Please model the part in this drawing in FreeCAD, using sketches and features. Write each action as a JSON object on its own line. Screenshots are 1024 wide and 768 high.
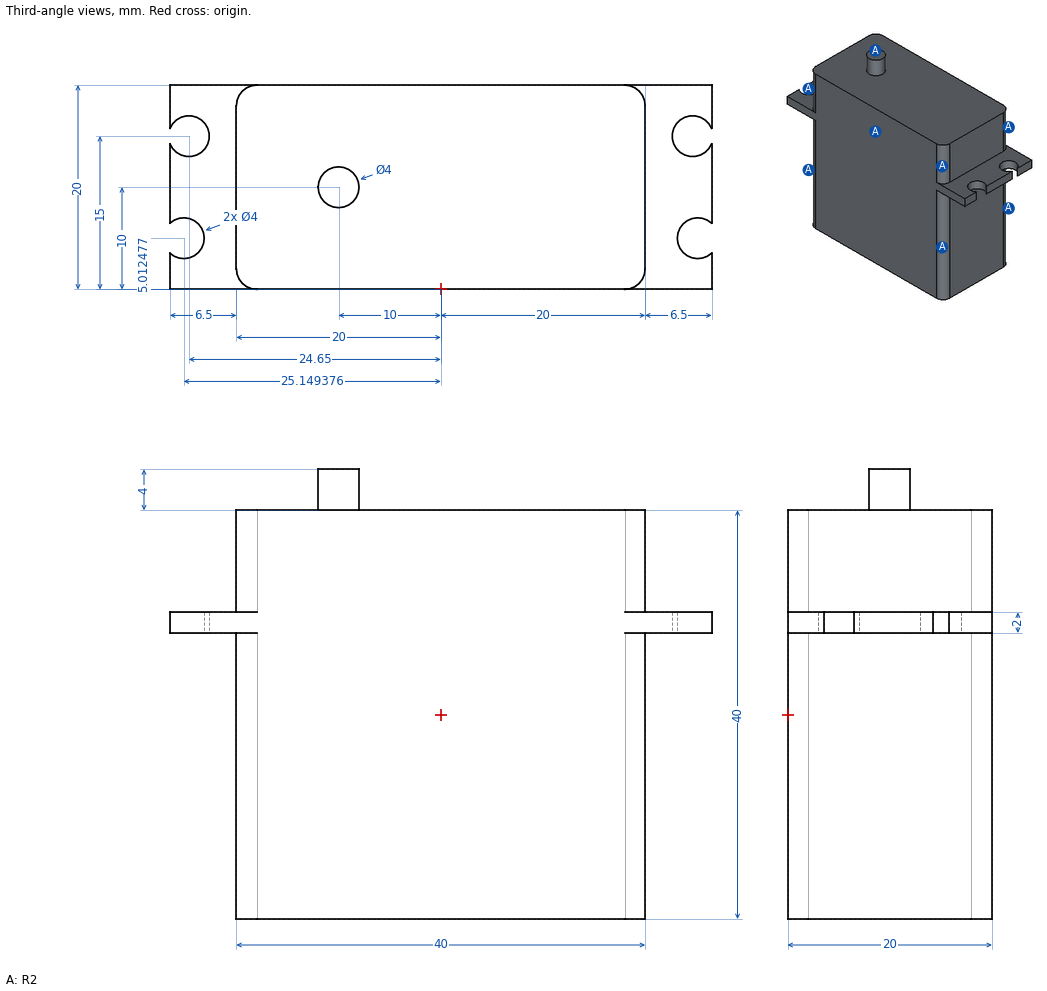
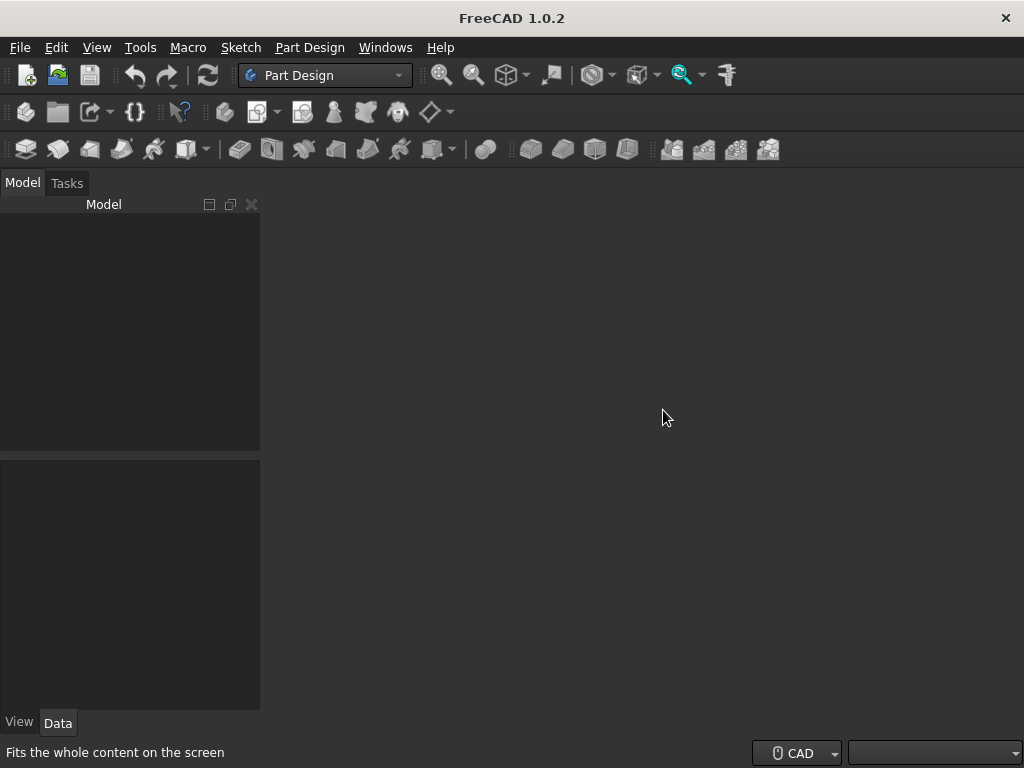
{"action": "key", "text": "ctrl+n"}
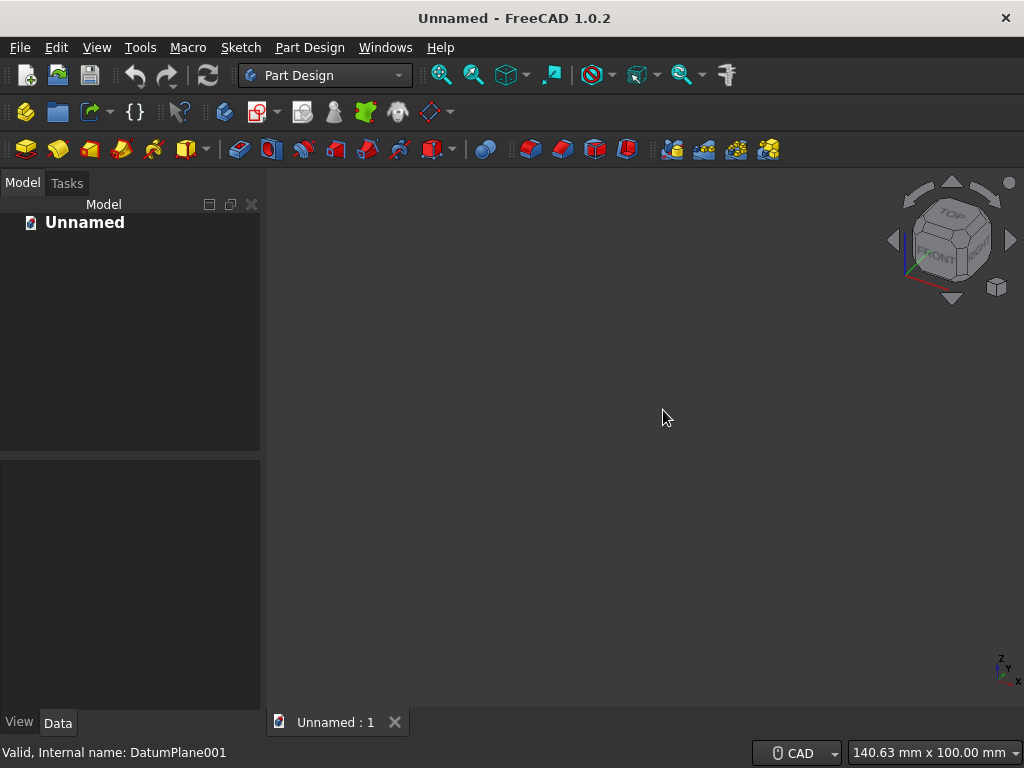
{"action": "left_click", "coordinate": [258, 112]}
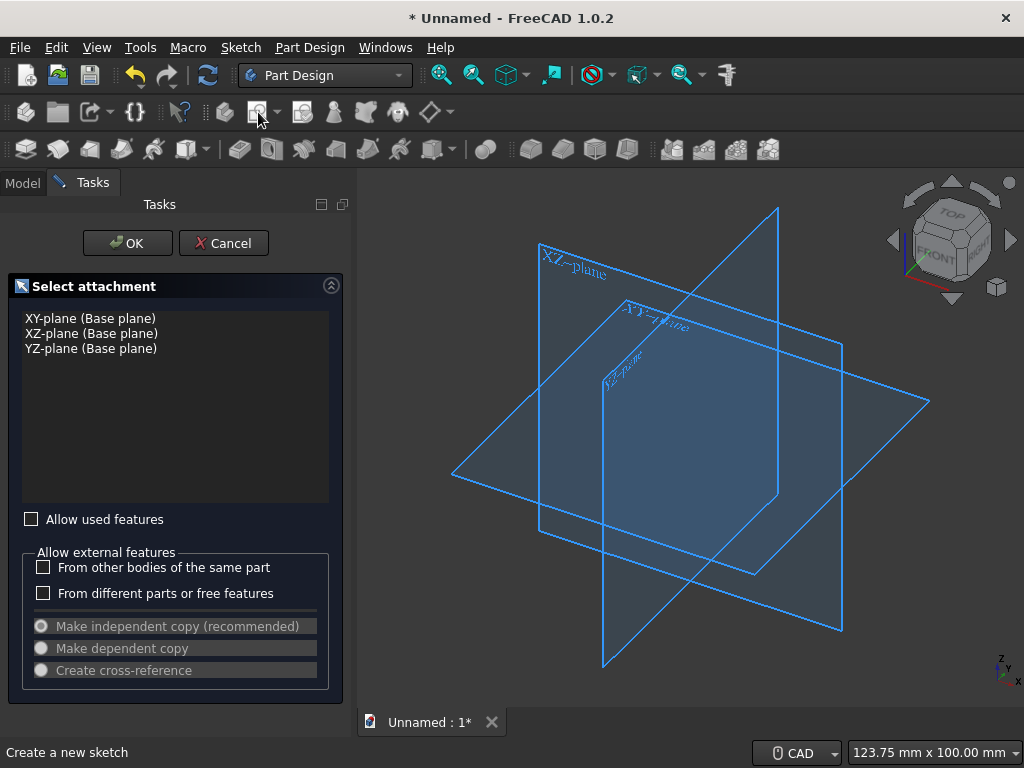
{"action": "left_click", "coordinate": [82, 334]}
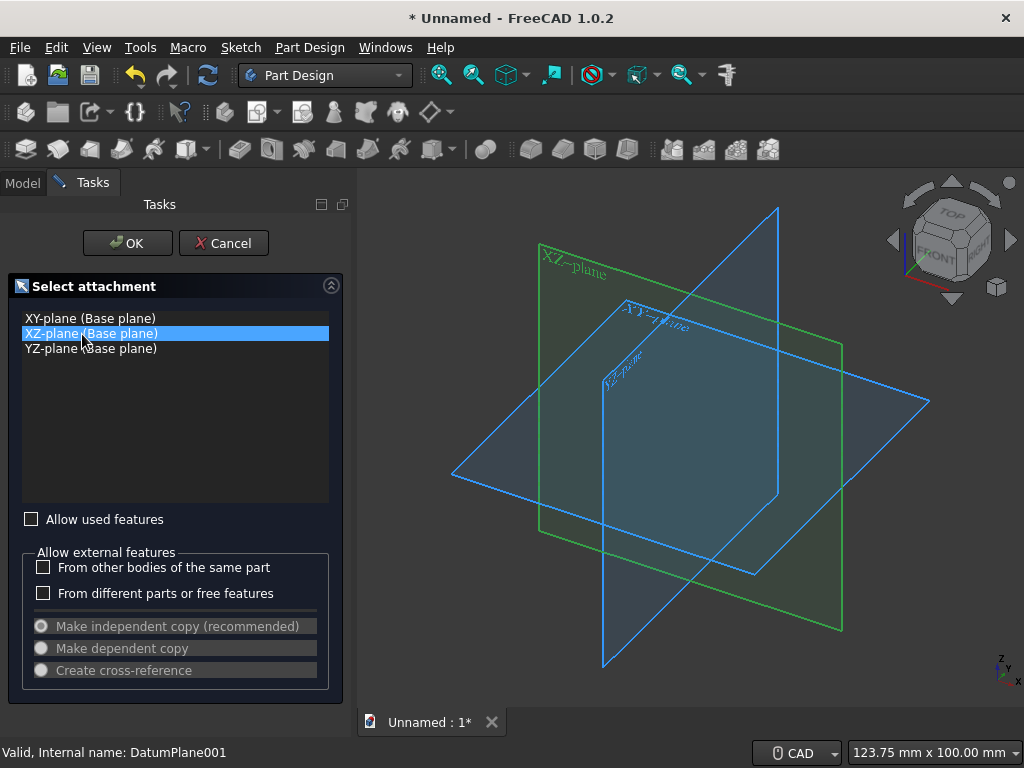
{"action": "left_click", "coordinate": [128, 243]}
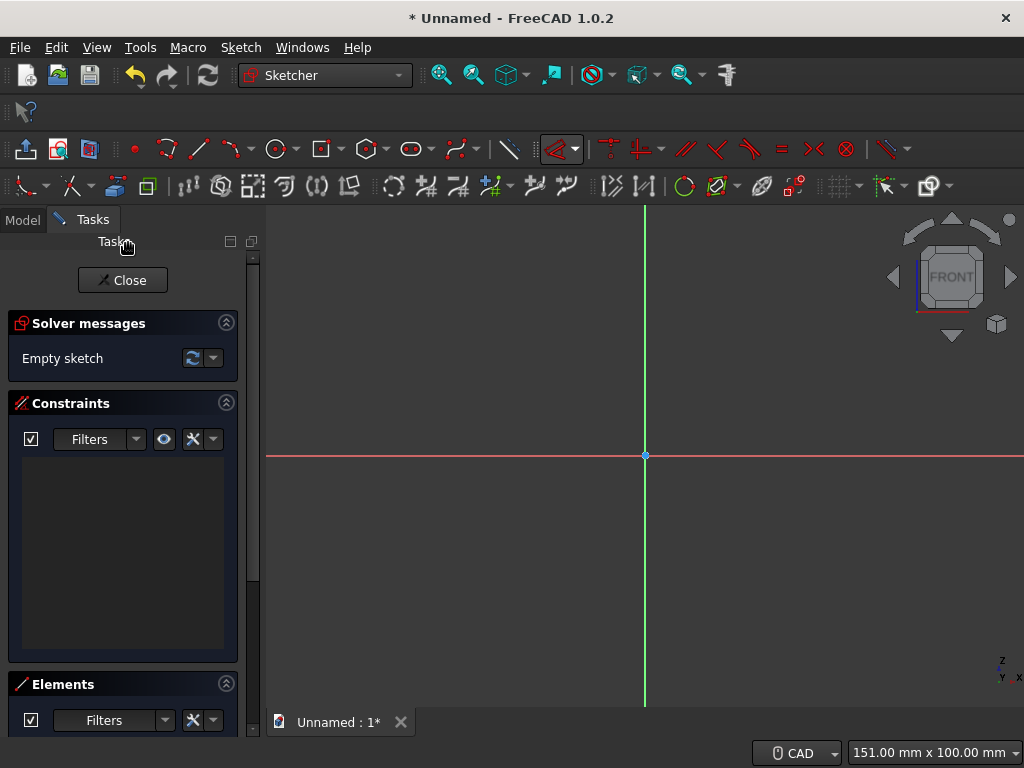
{"action": "scroll", "coordinate": [784, 456], "scroll_direction": "up", "scroll_amount": 2}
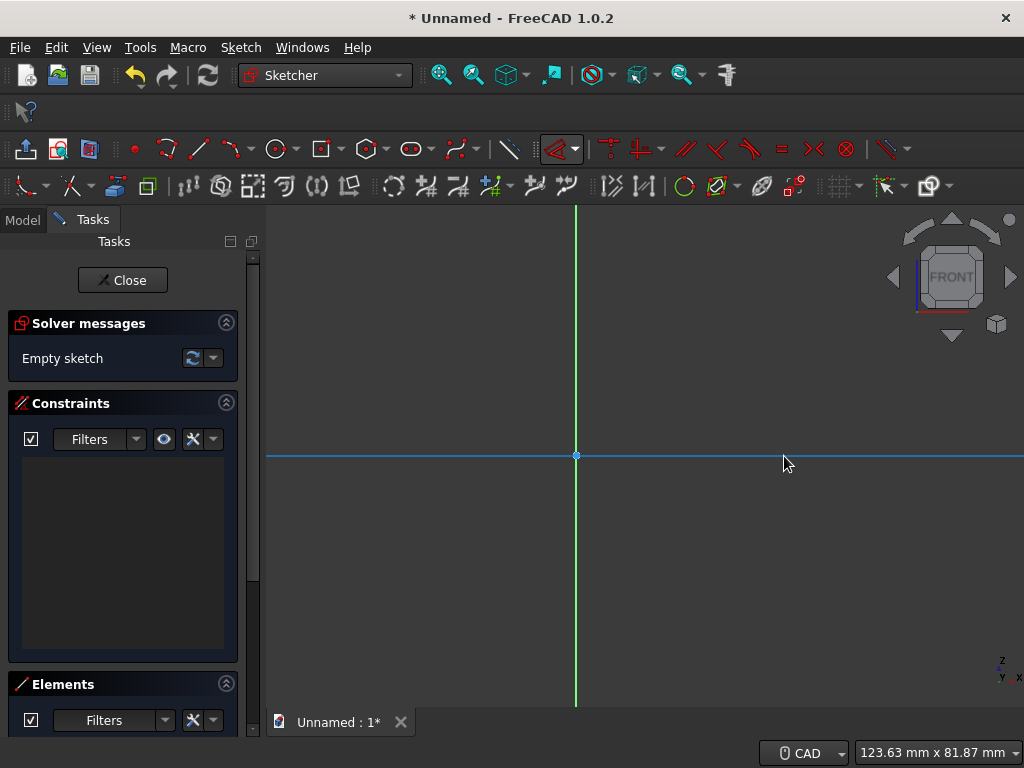
{"action": "left_click", "coordinate": [322, 150]}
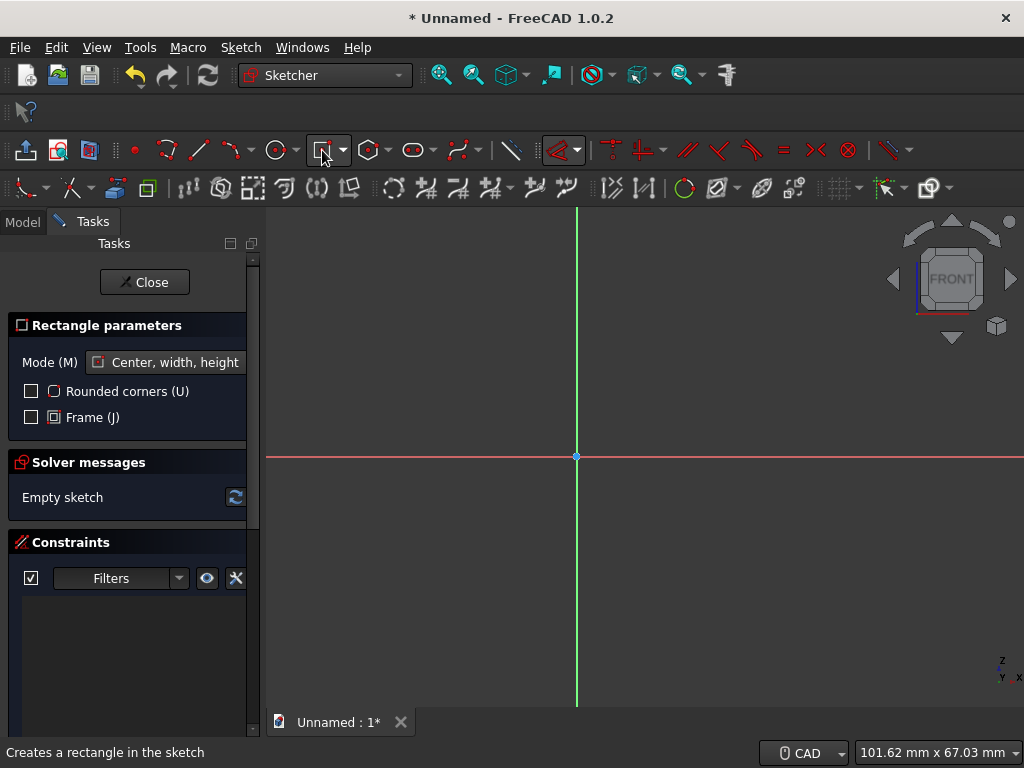
{"action": "left_click", "coordinate": [577, 457]}
{"action": "left_click", "coordinate": [726, 308]}
{"action": "key", "text": "Escape"}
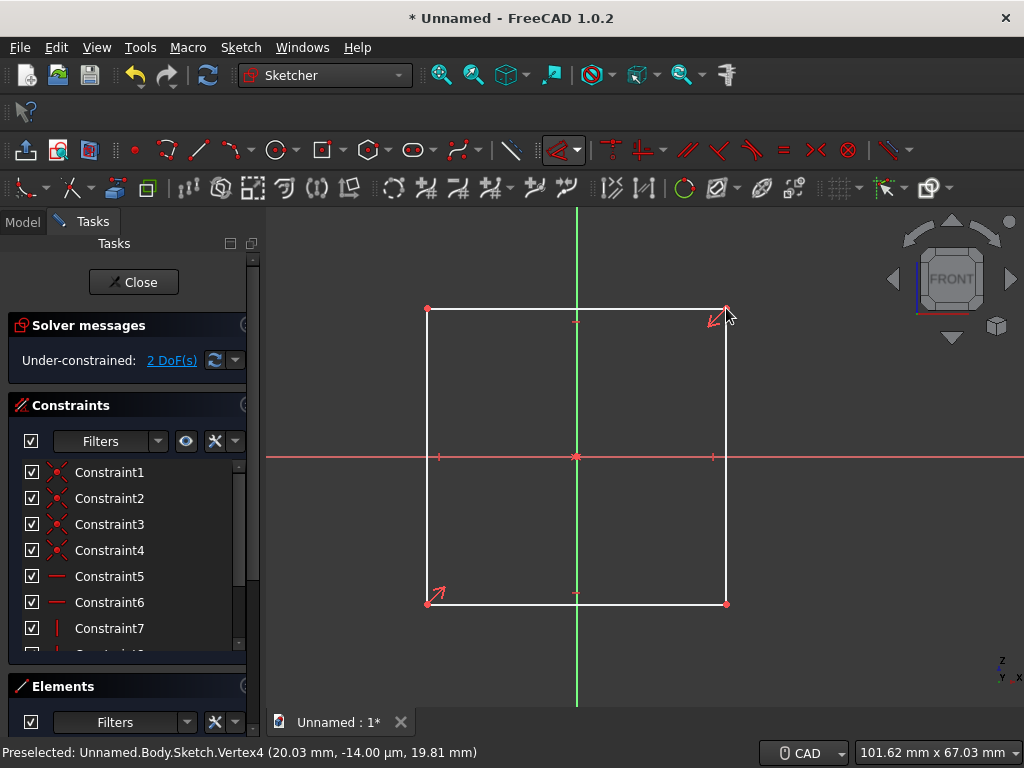
{"action": "left_click", "coordinate": [517, 605]}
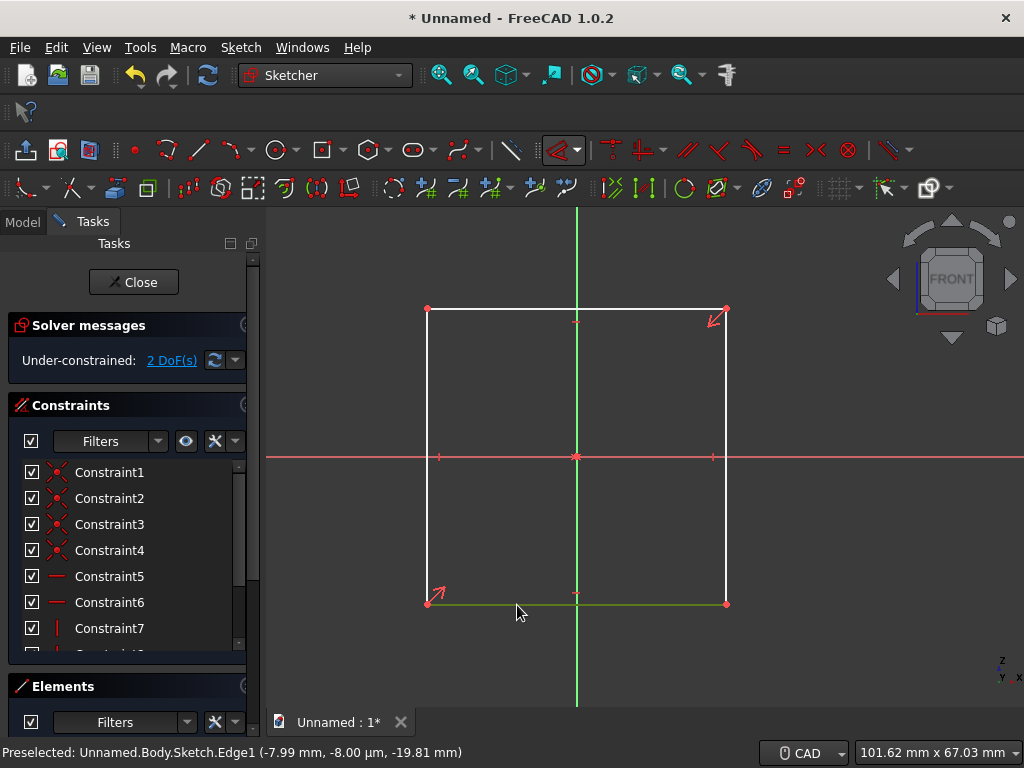
{"action": "key", "text": "l"}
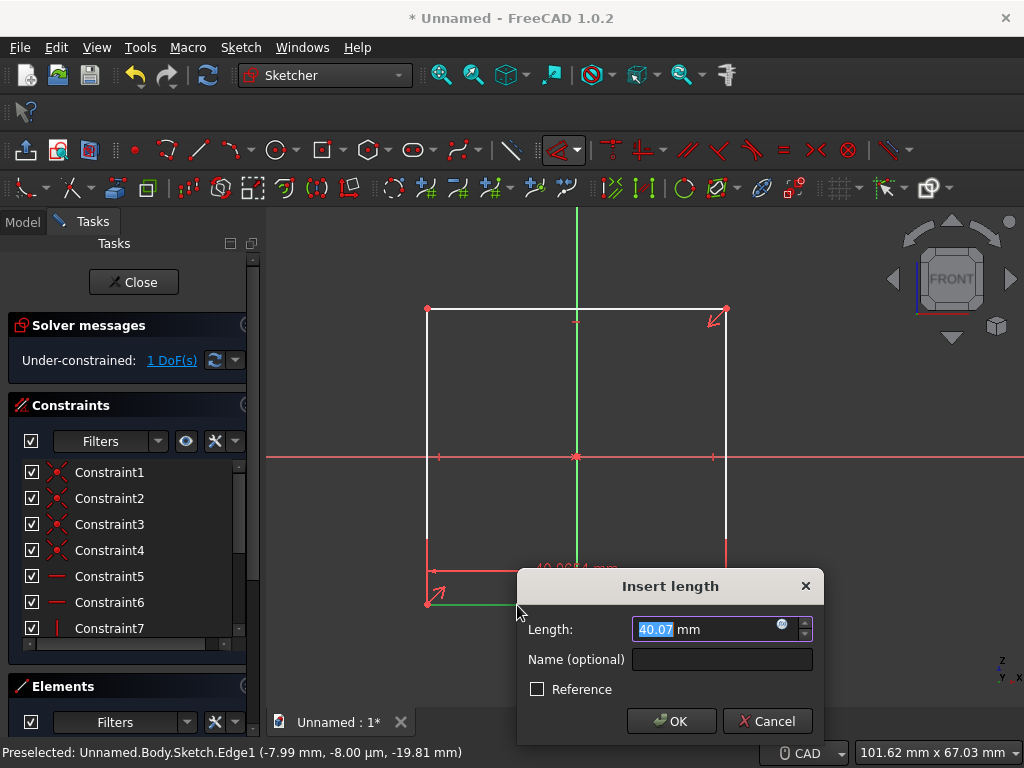
{"action": "type", "text": "40"}
{"action": "key", "text": "Return"}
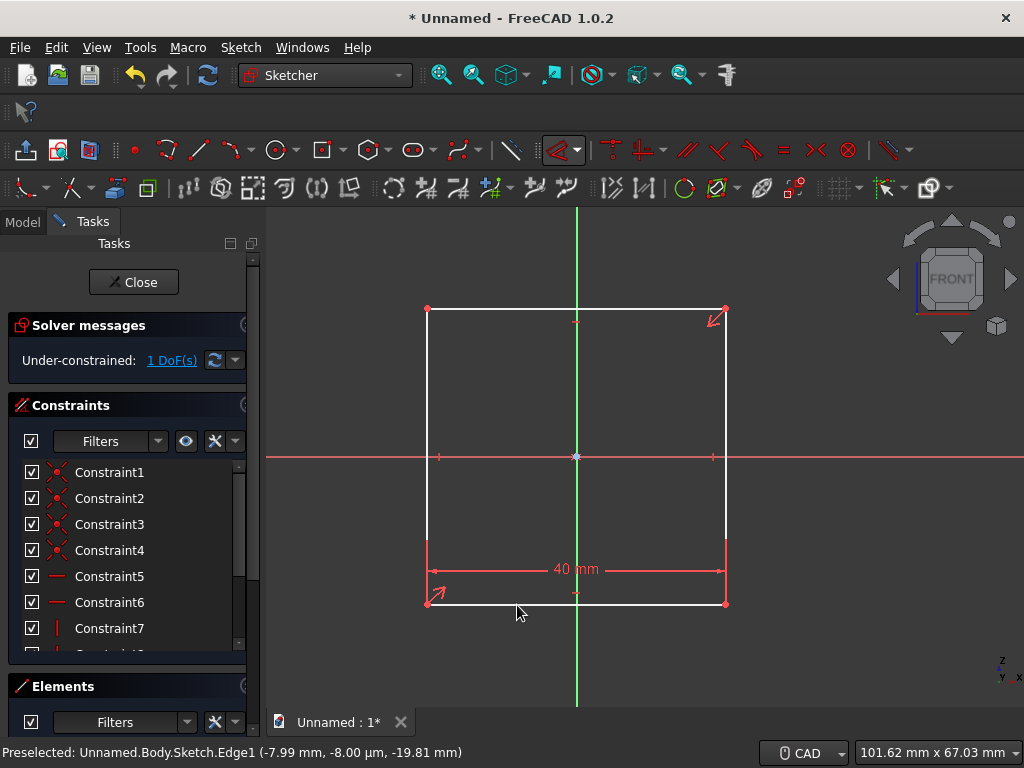
{"action": "left_click", "coordinate": [726, 516]}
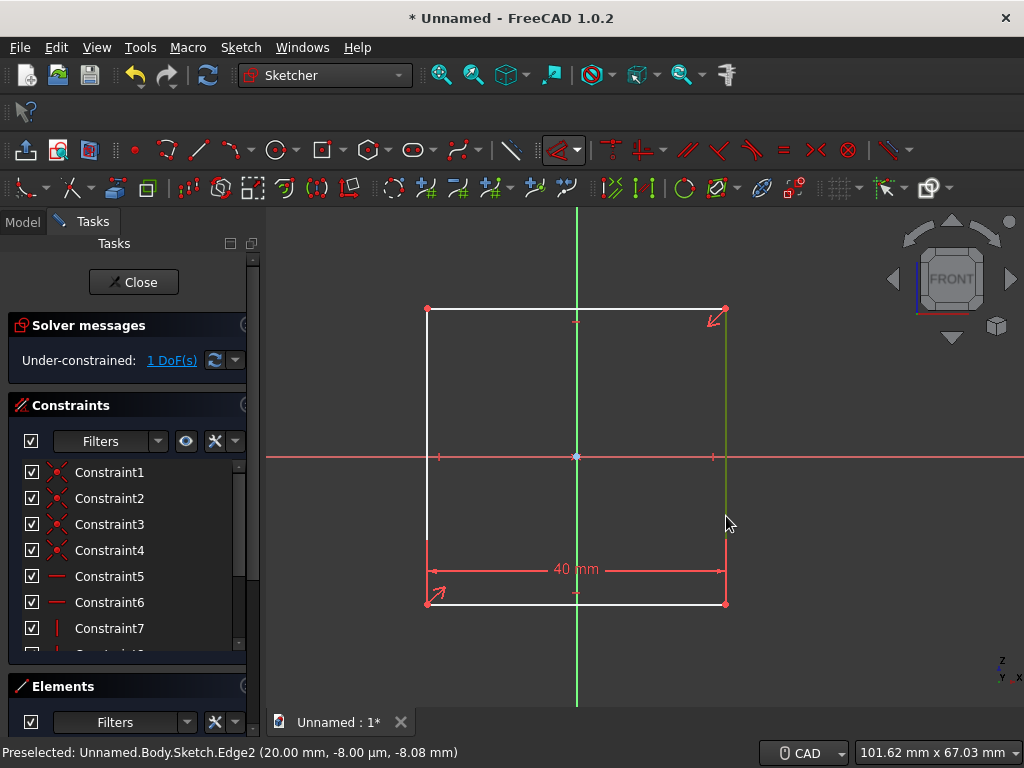
{"action": "key", "text": "i"}